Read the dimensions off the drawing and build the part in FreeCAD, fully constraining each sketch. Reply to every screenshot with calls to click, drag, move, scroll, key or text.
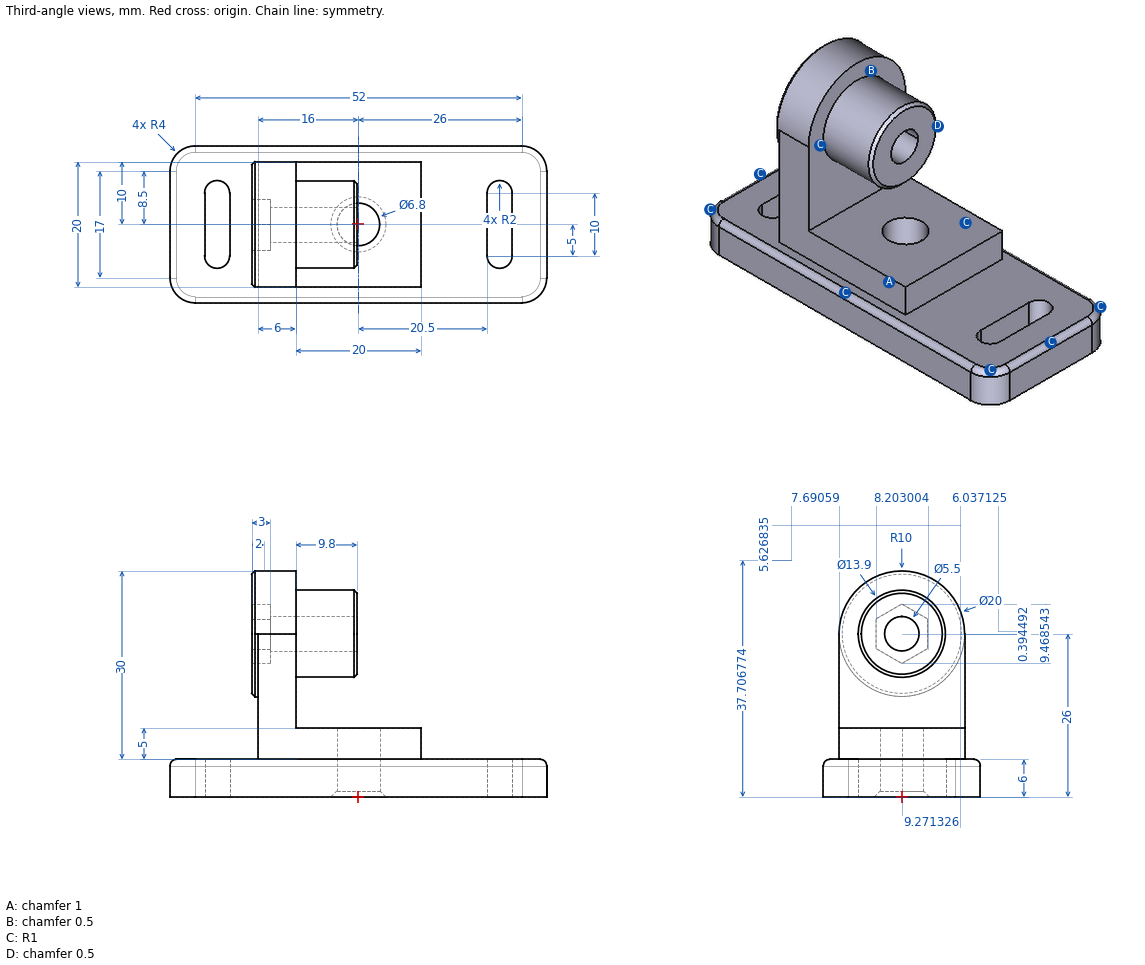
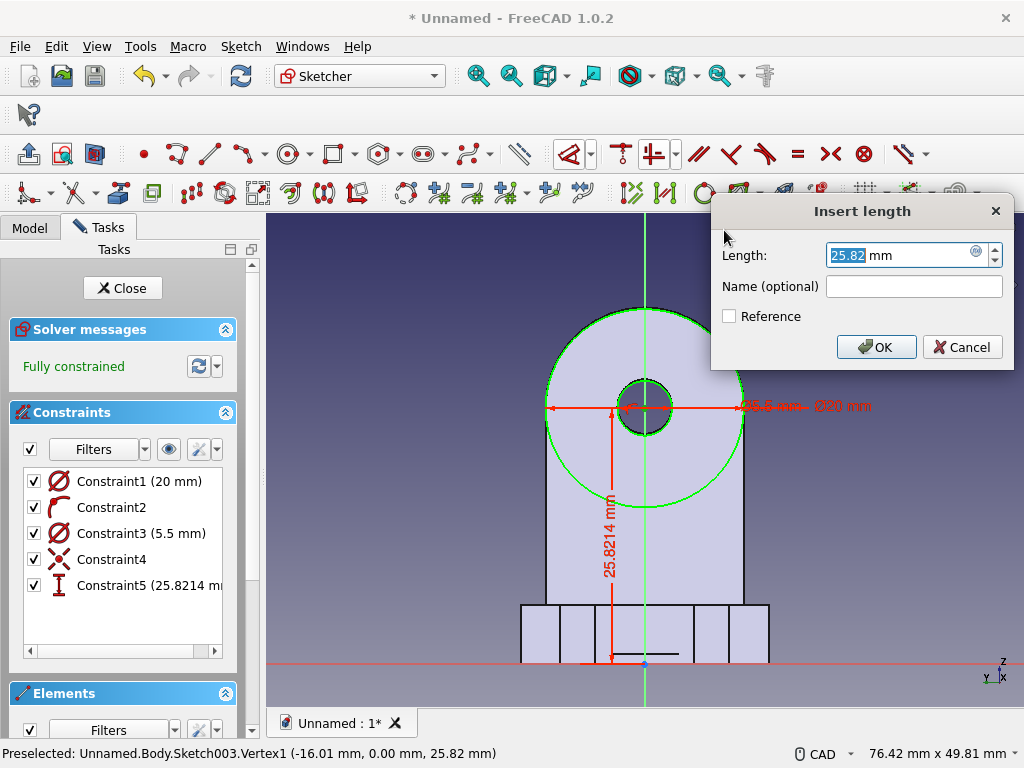
text(26)
key(Return)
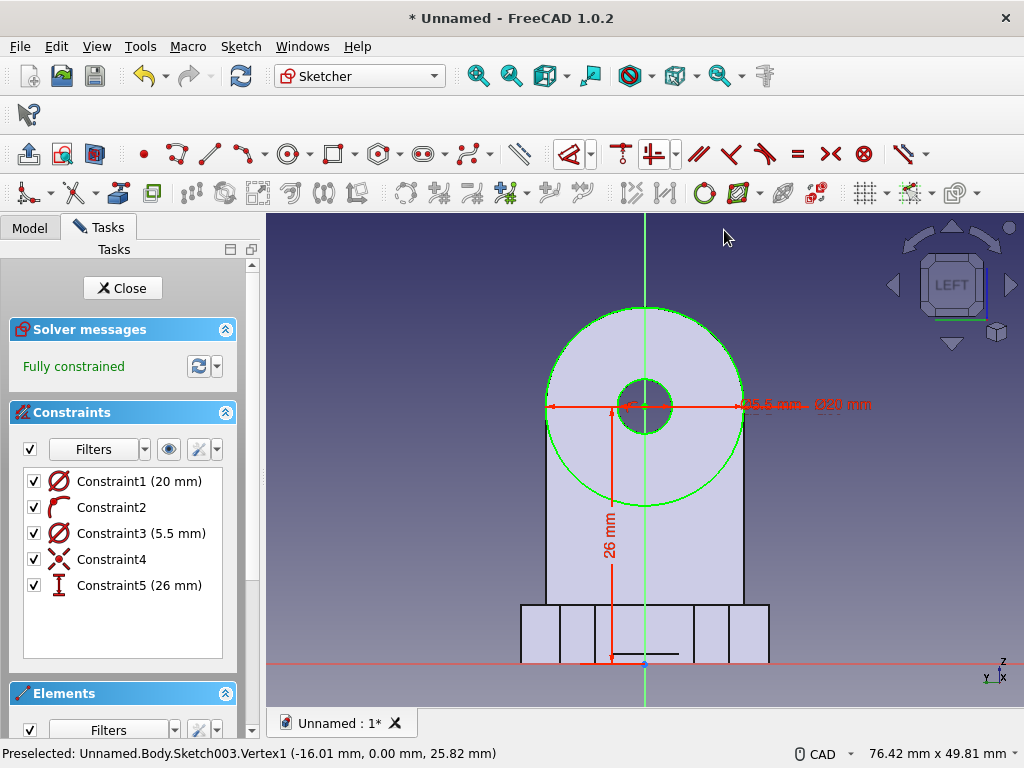
click(123, 288)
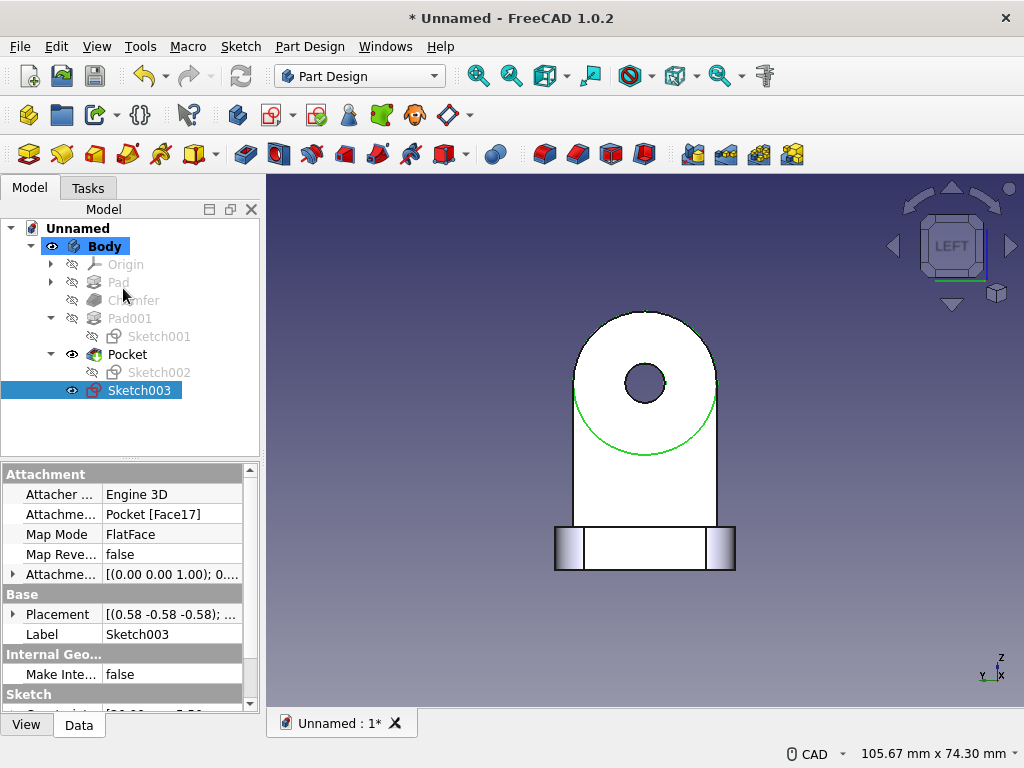
click(29, 154)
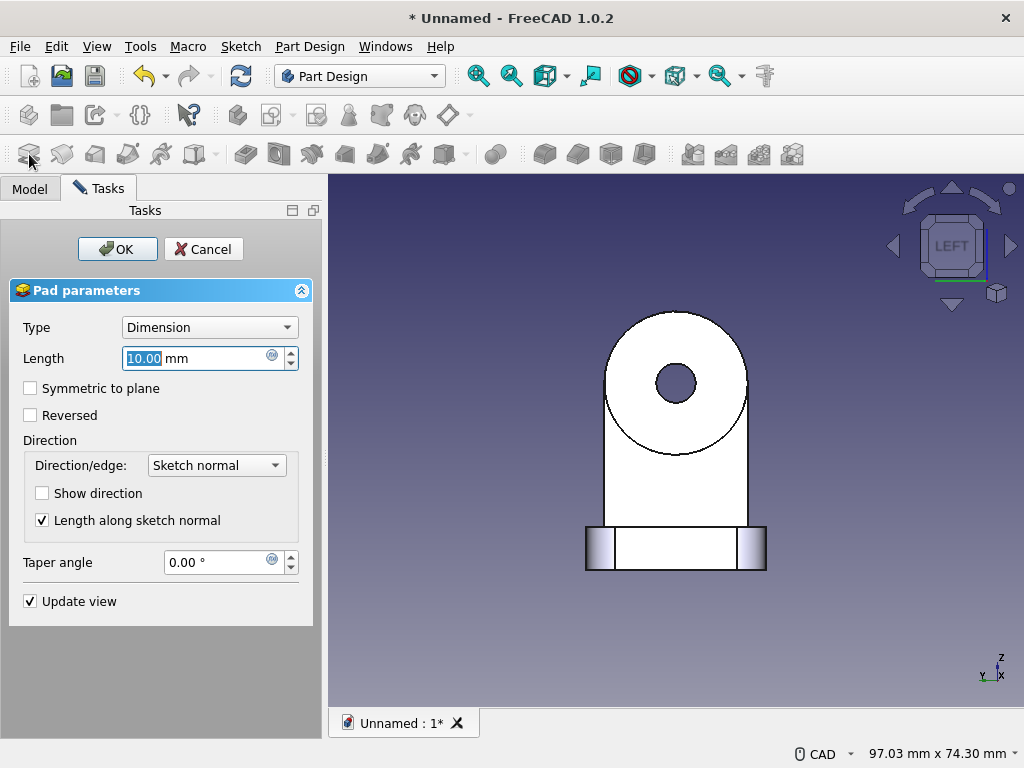
text(2)
key(Tab)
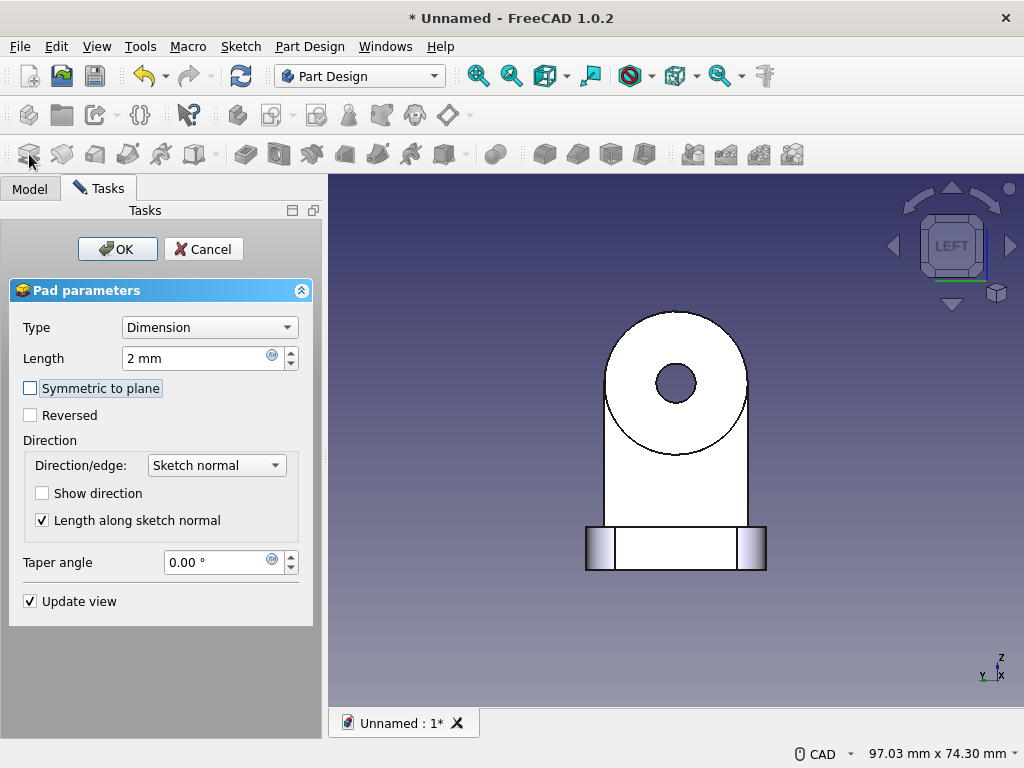
click(31, 388)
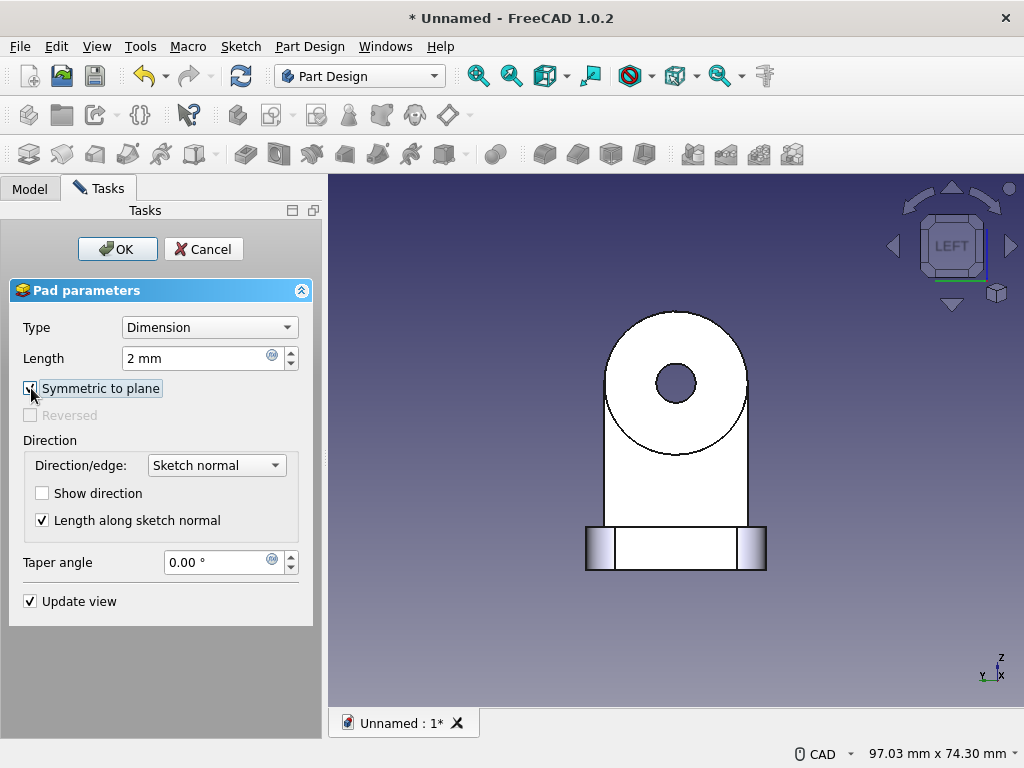
click(118, 249)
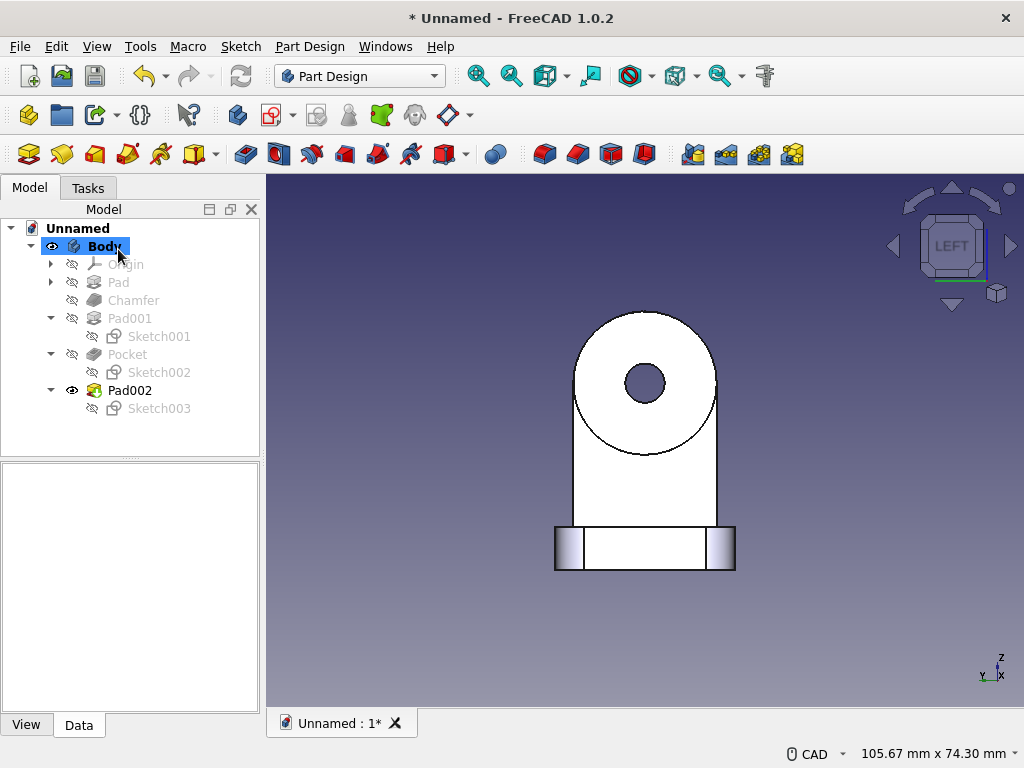
click(573, 382)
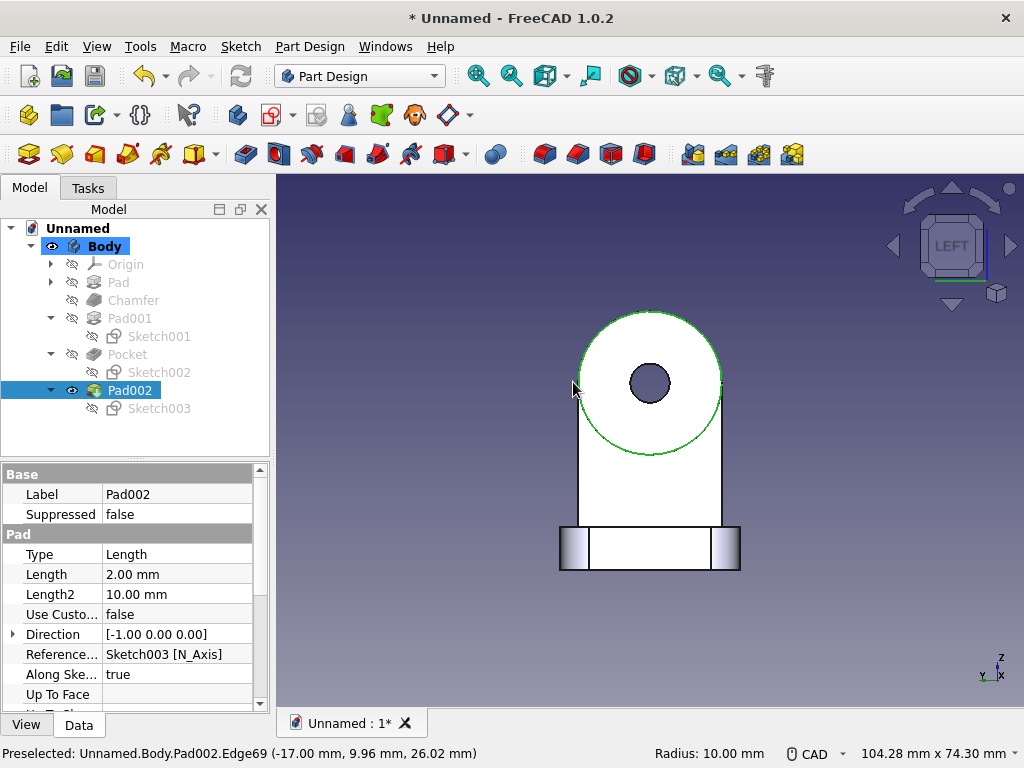
click(578, 154)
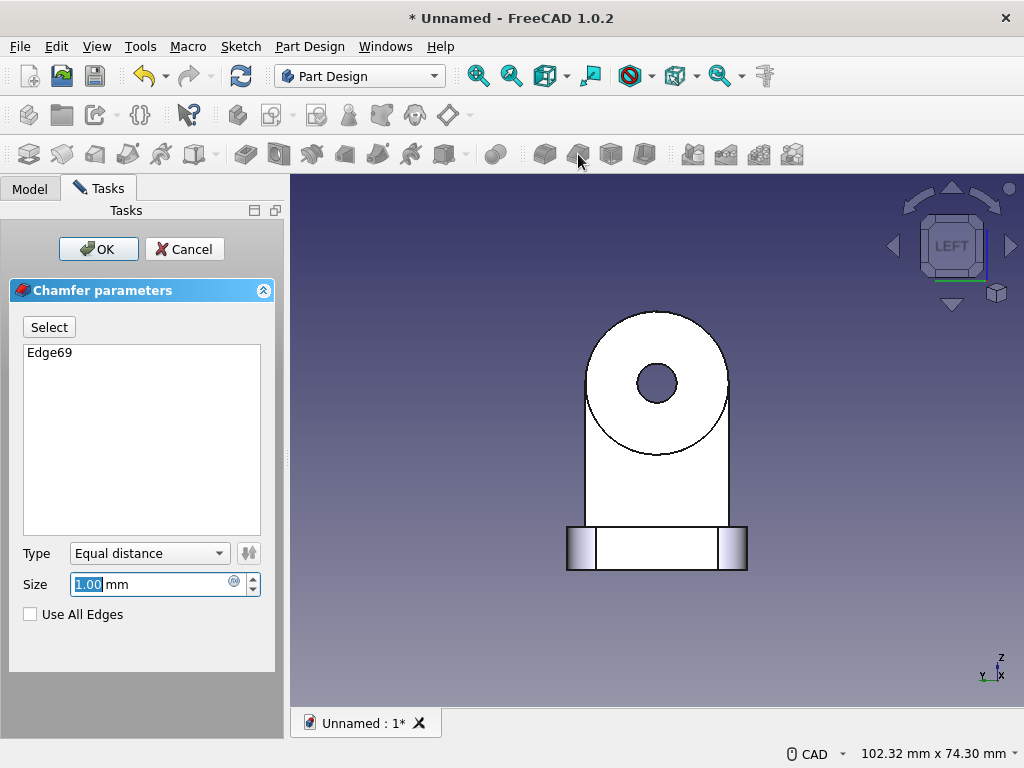
text(0.5)
key(Tab)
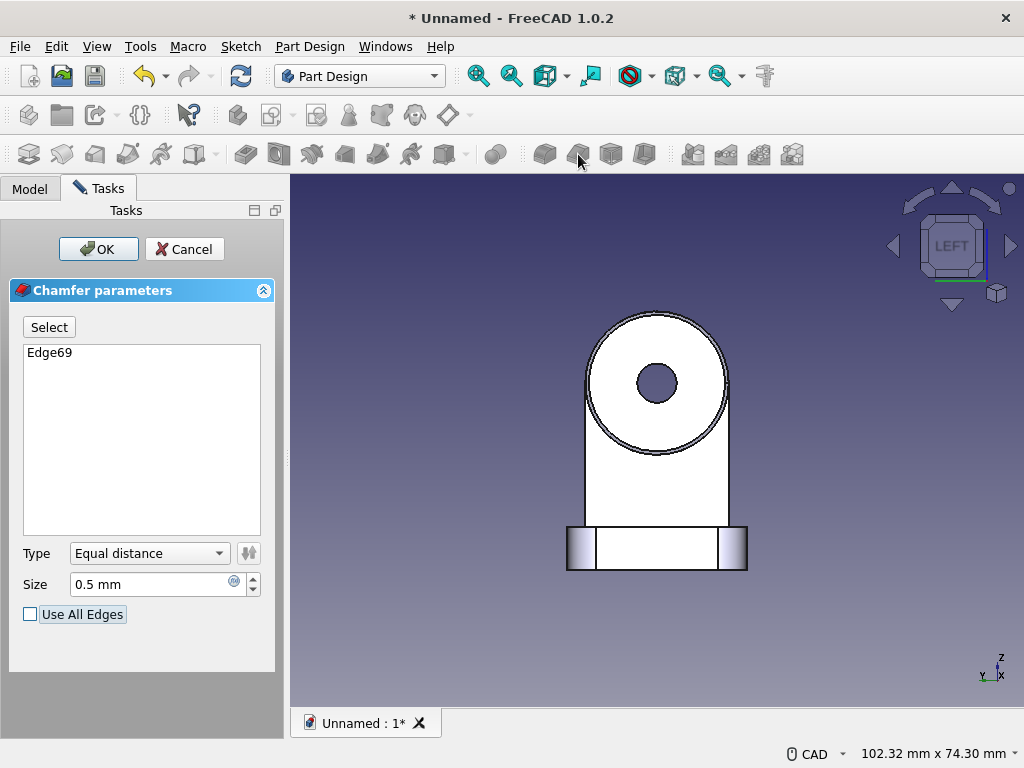
click(99, 249)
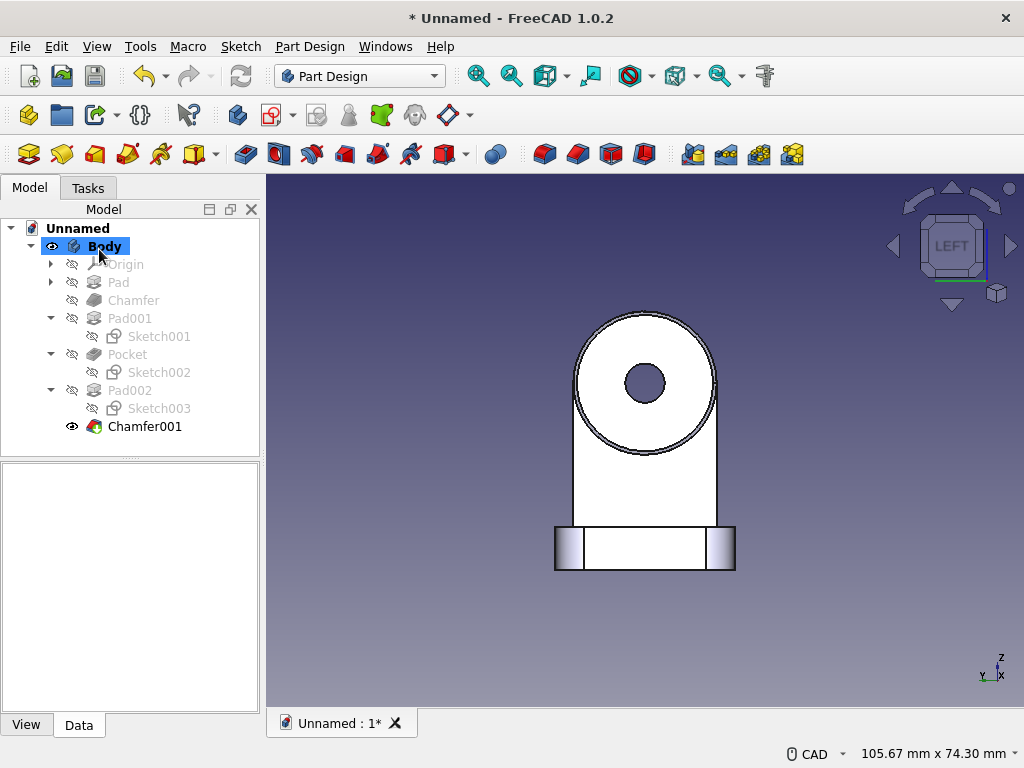
click(564, 526)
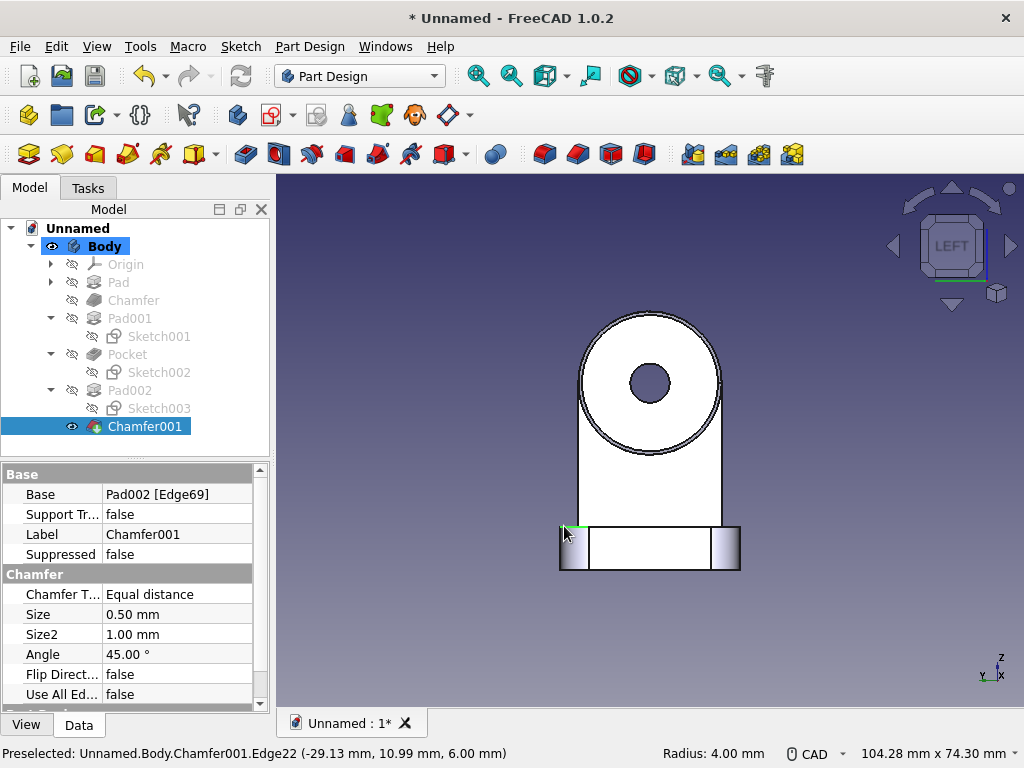
click(650, 526, ctrl)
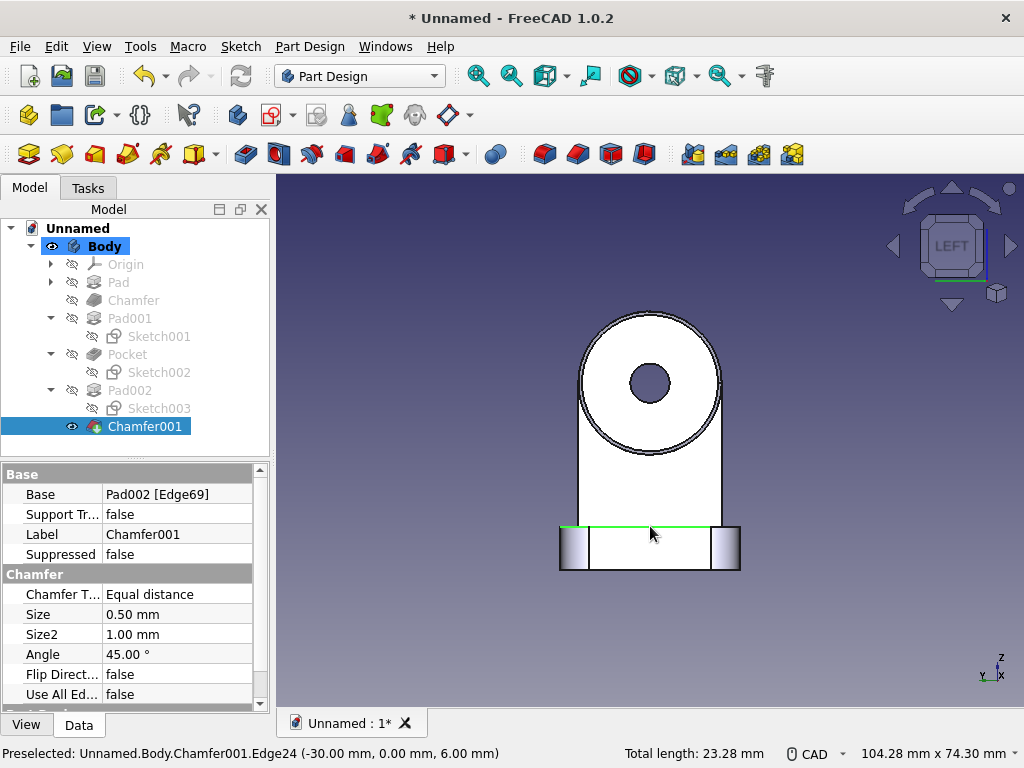
click(731, 526, ctrl)